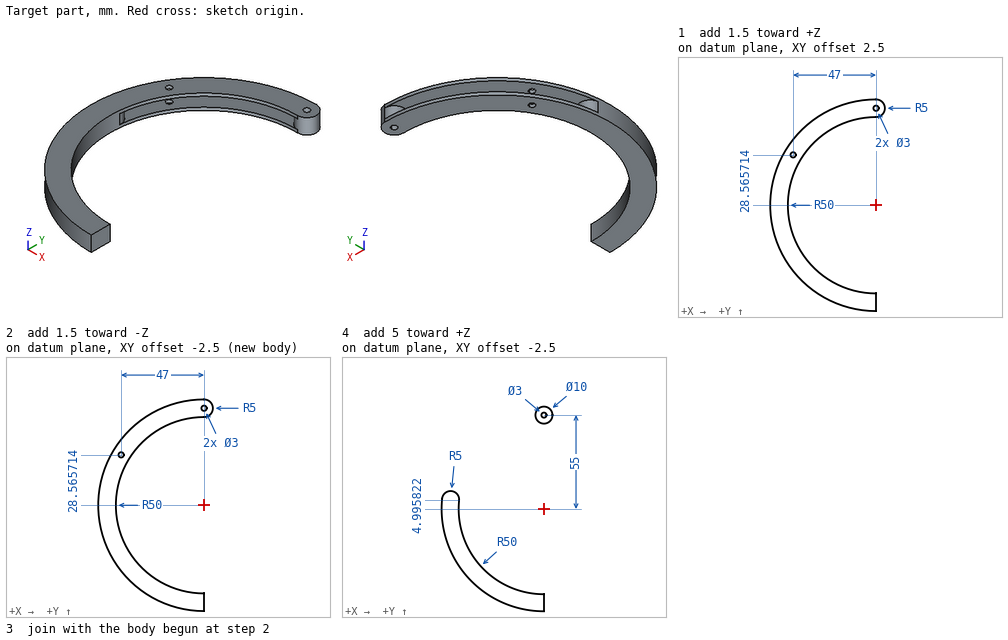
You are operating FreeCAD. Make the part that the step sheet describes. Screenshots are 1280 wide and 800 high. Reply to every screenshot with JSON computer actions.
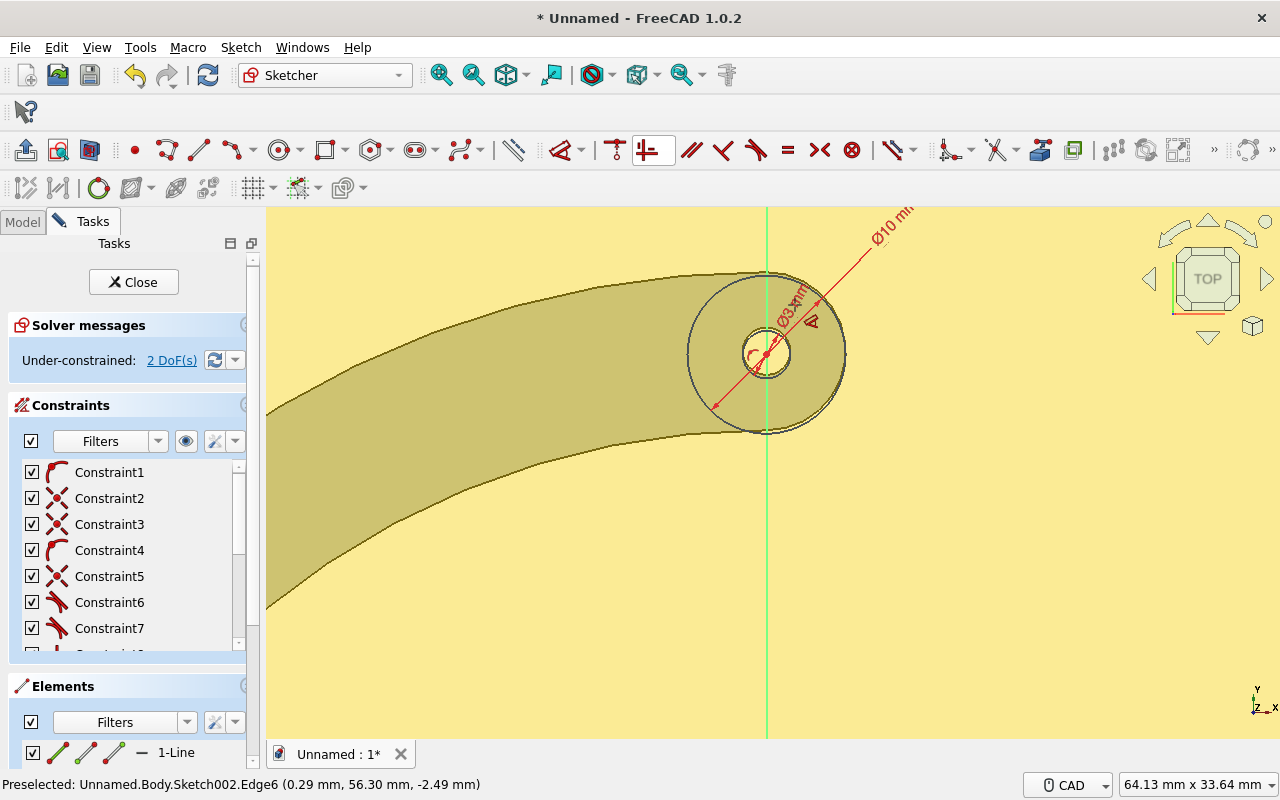
{"action": "scroll", "coordinate": [778, 325], "scroll_direction": "down", "scroll_amount": 9}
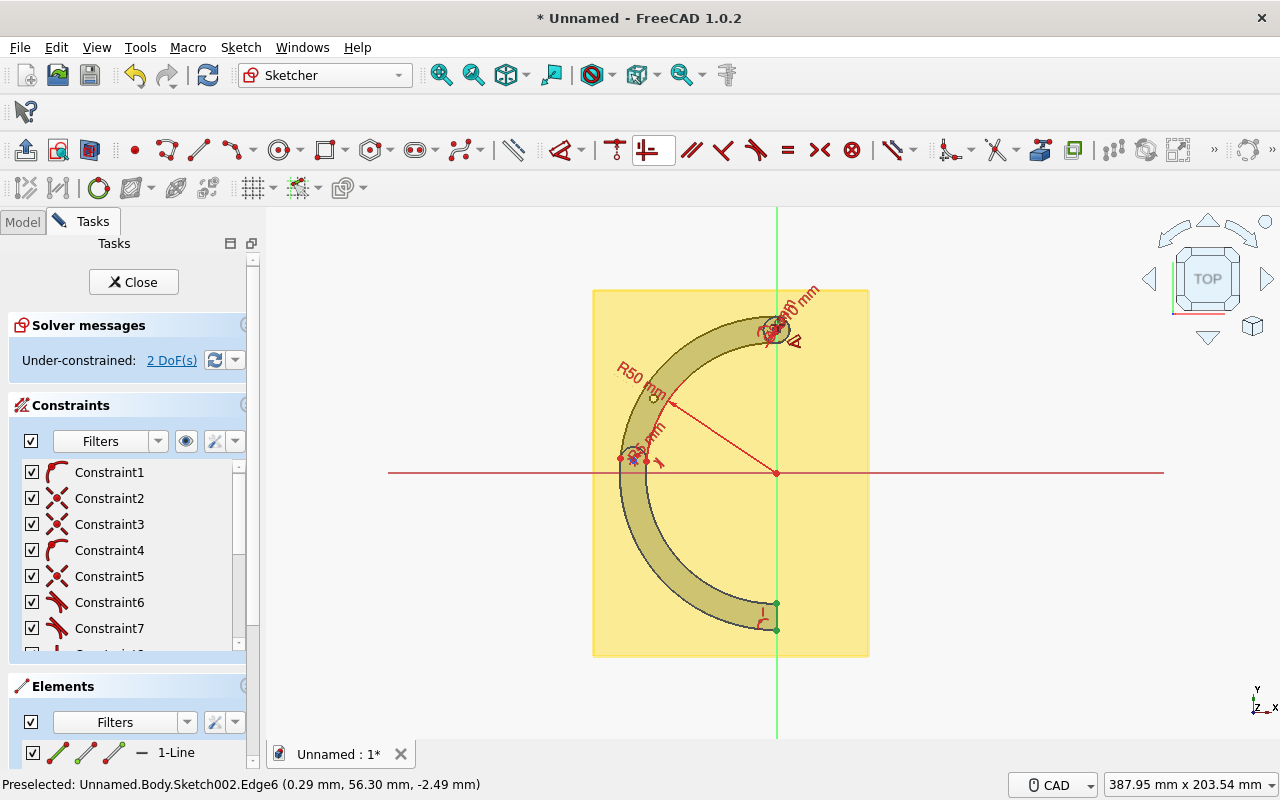
{"action": "left_click", "coordinate": [777, 330]}
{"action": "left_click", "coordinate": [811, 402]}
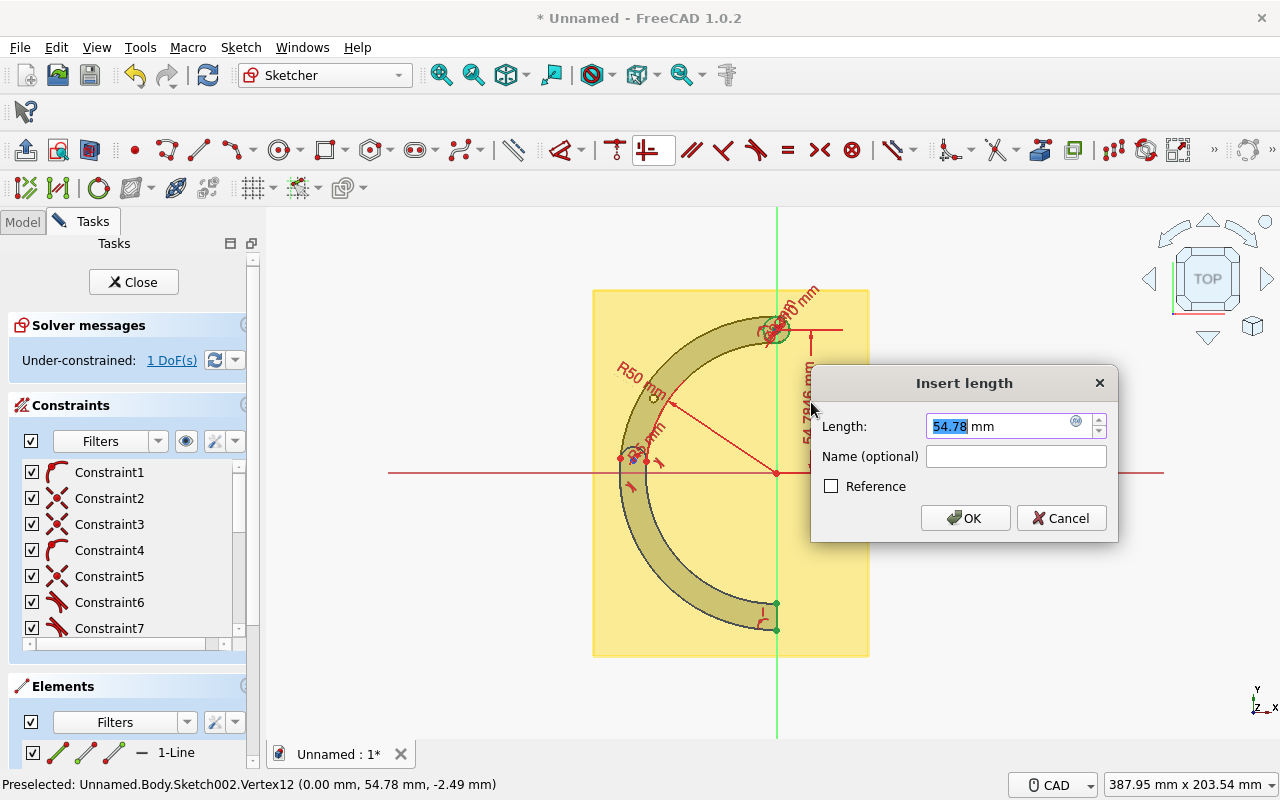
{"action": "type", "text": "55"}
{"action": "key", "text": "Return"}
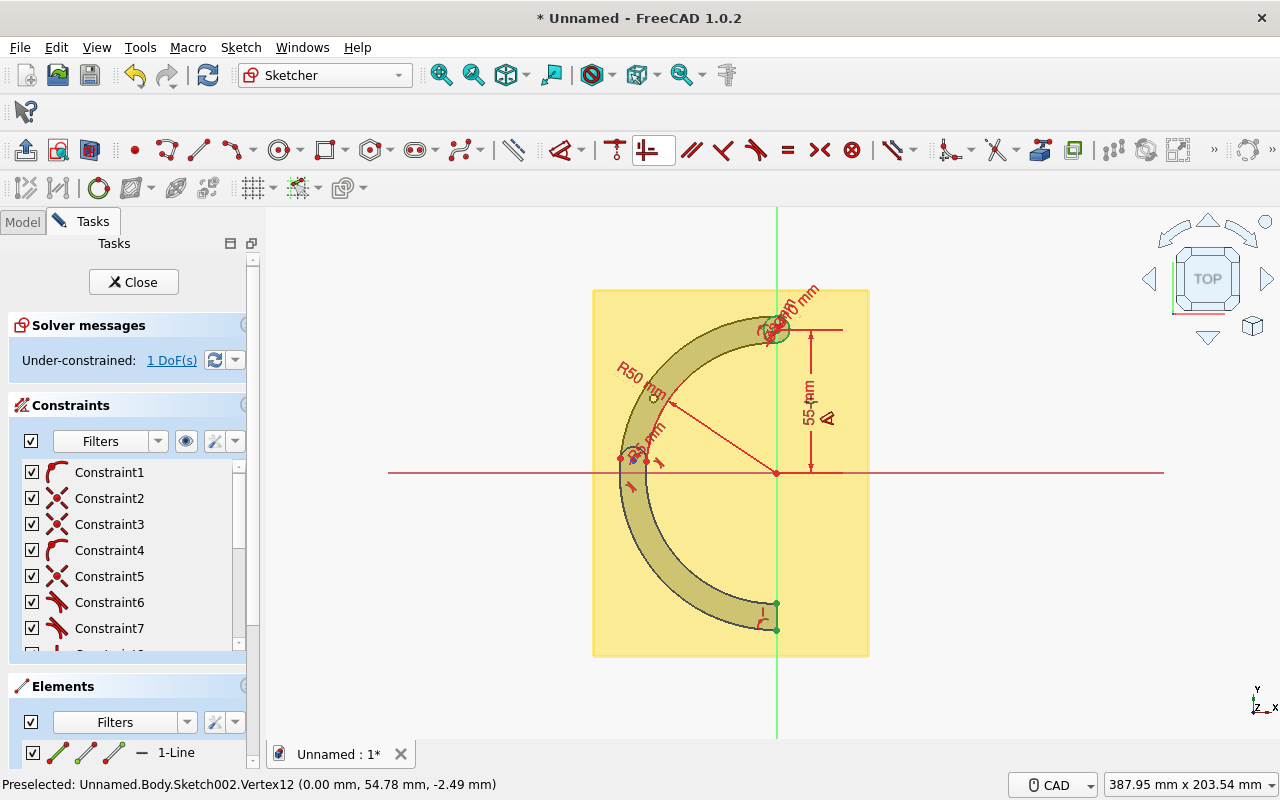
{"action": "scroll", "coordinate": [646, 461], "scroll_direction": "up", "scroll_amount": 6}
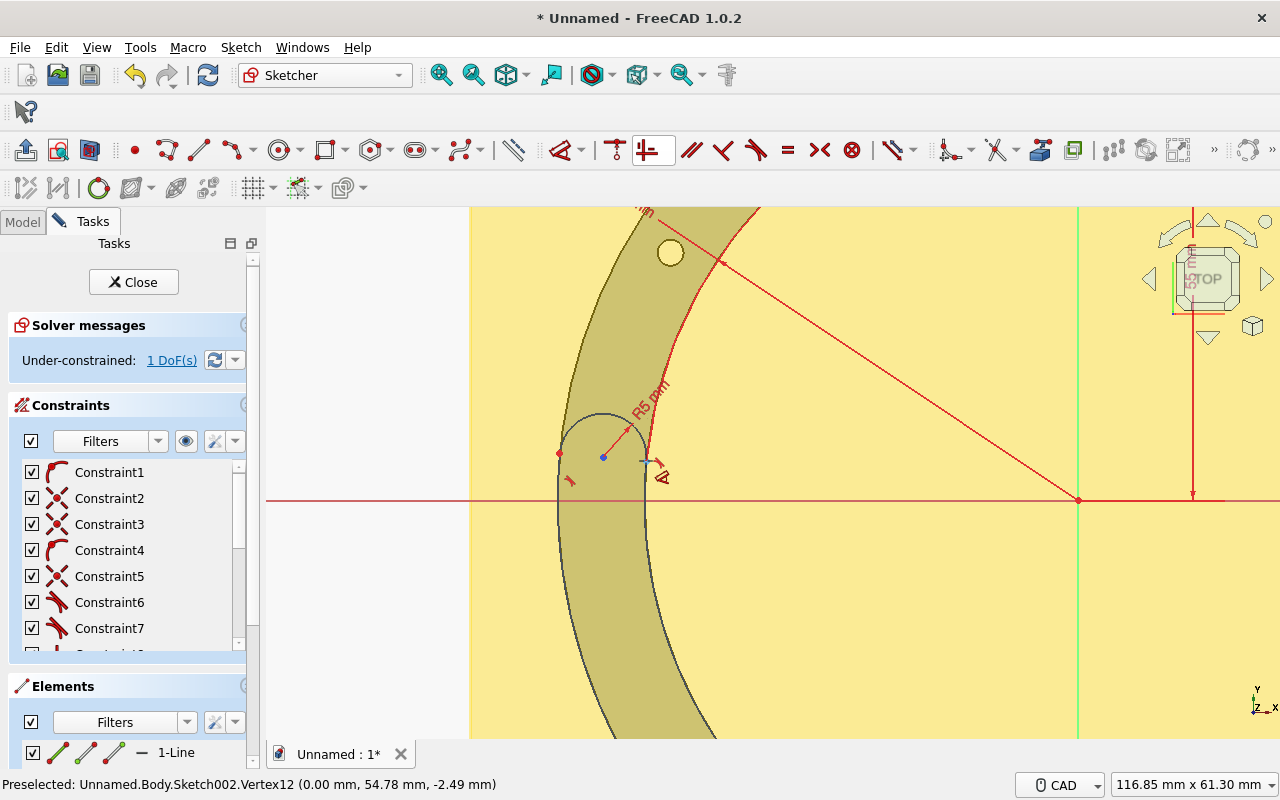
{"action": "left_click", "coordinate": [646, 461]}
{"action": "left_click", "coordinate": [1112, 481]}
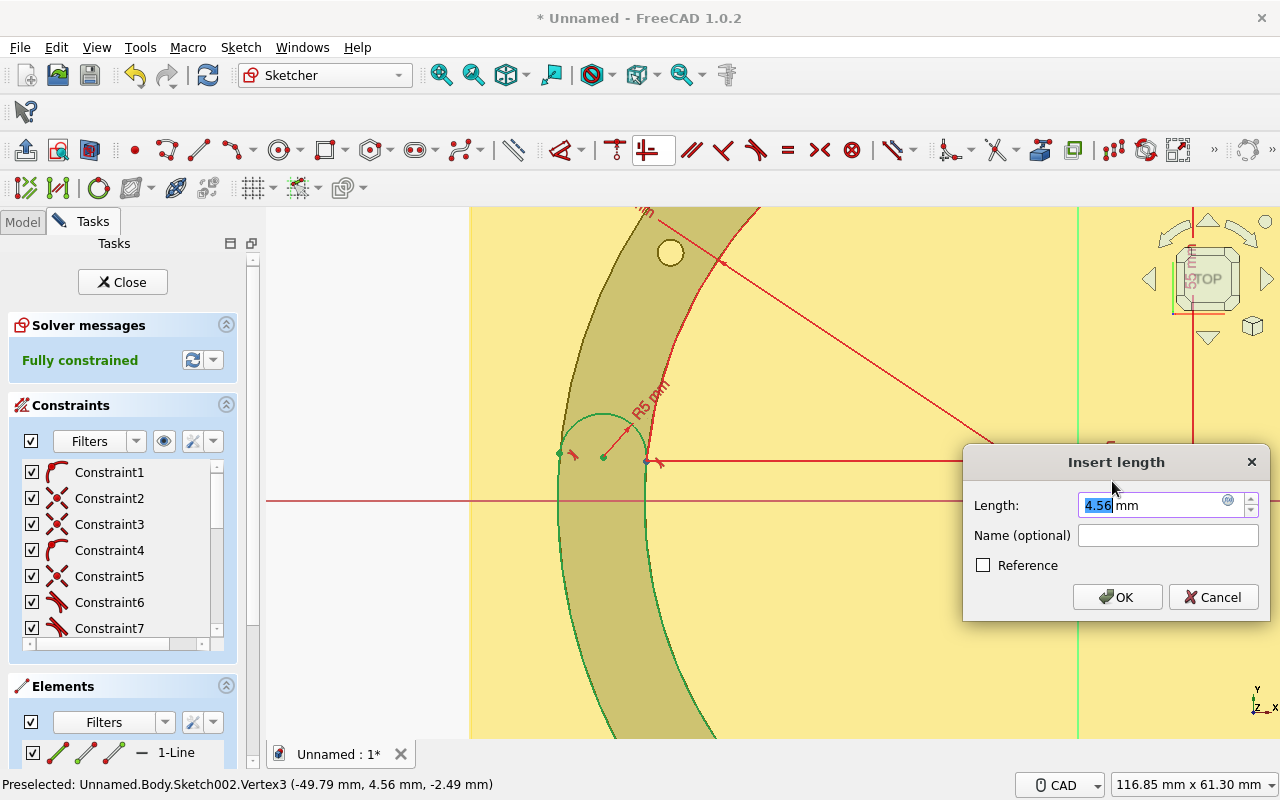
{"action": "type", "text": "4.995822"}
{"action": "key", "text": "Return"}
{"action": "key", "text": "Escape"}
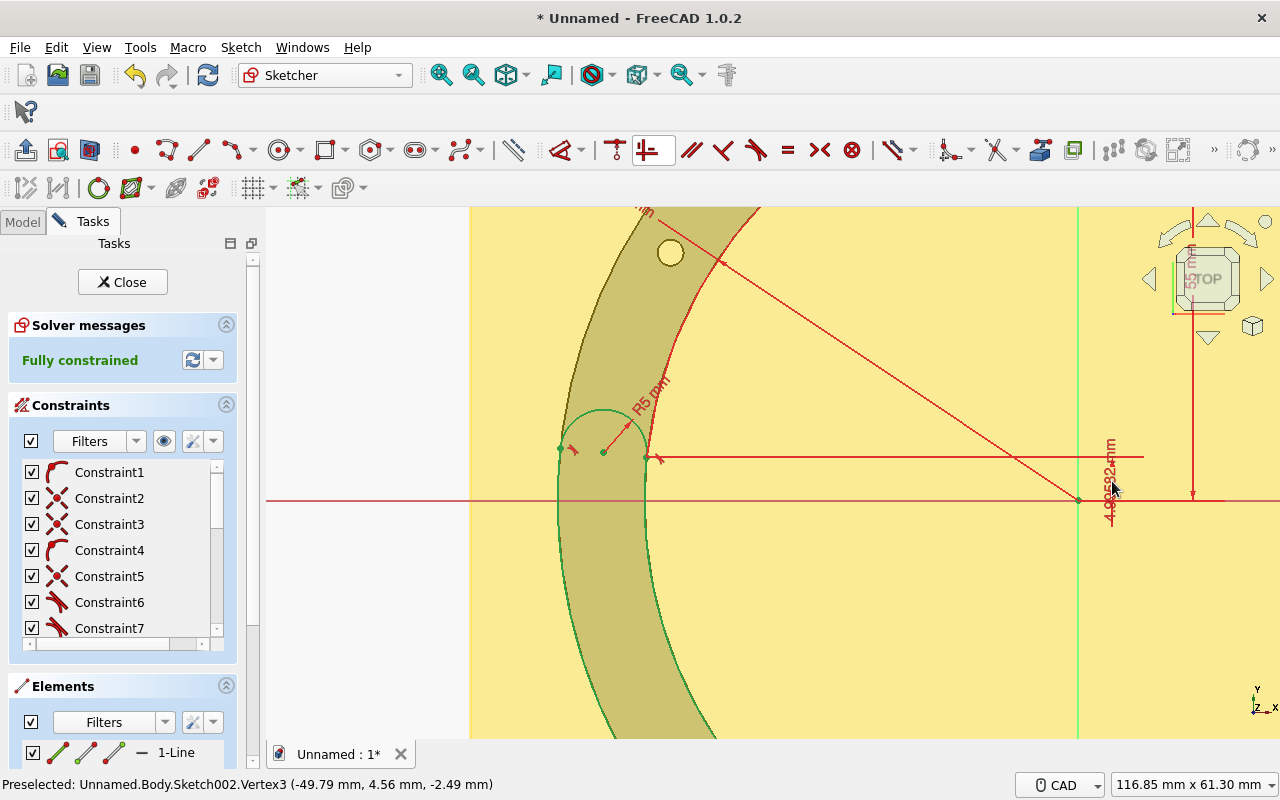
{"action": "left_click", "coordinate": [123, 282]}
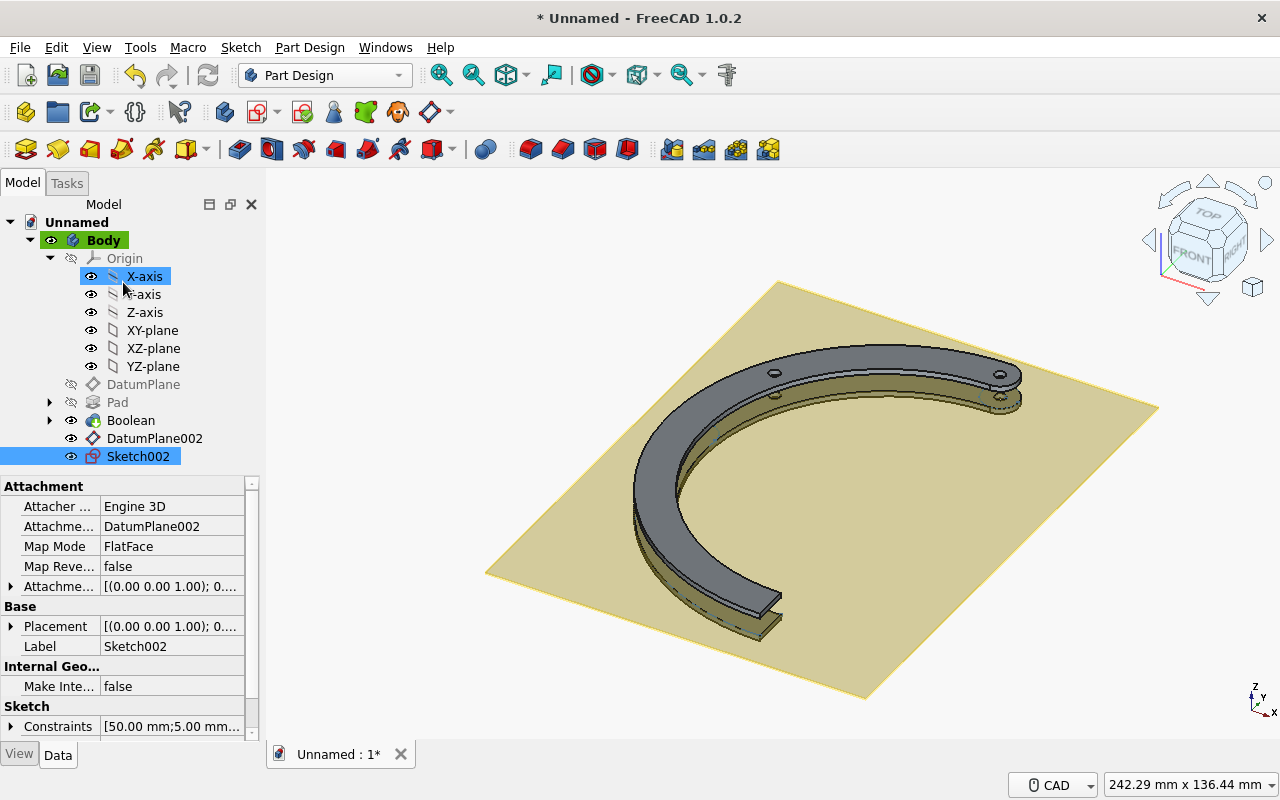
{"action": "left_click", "coordinate": [26, 150]}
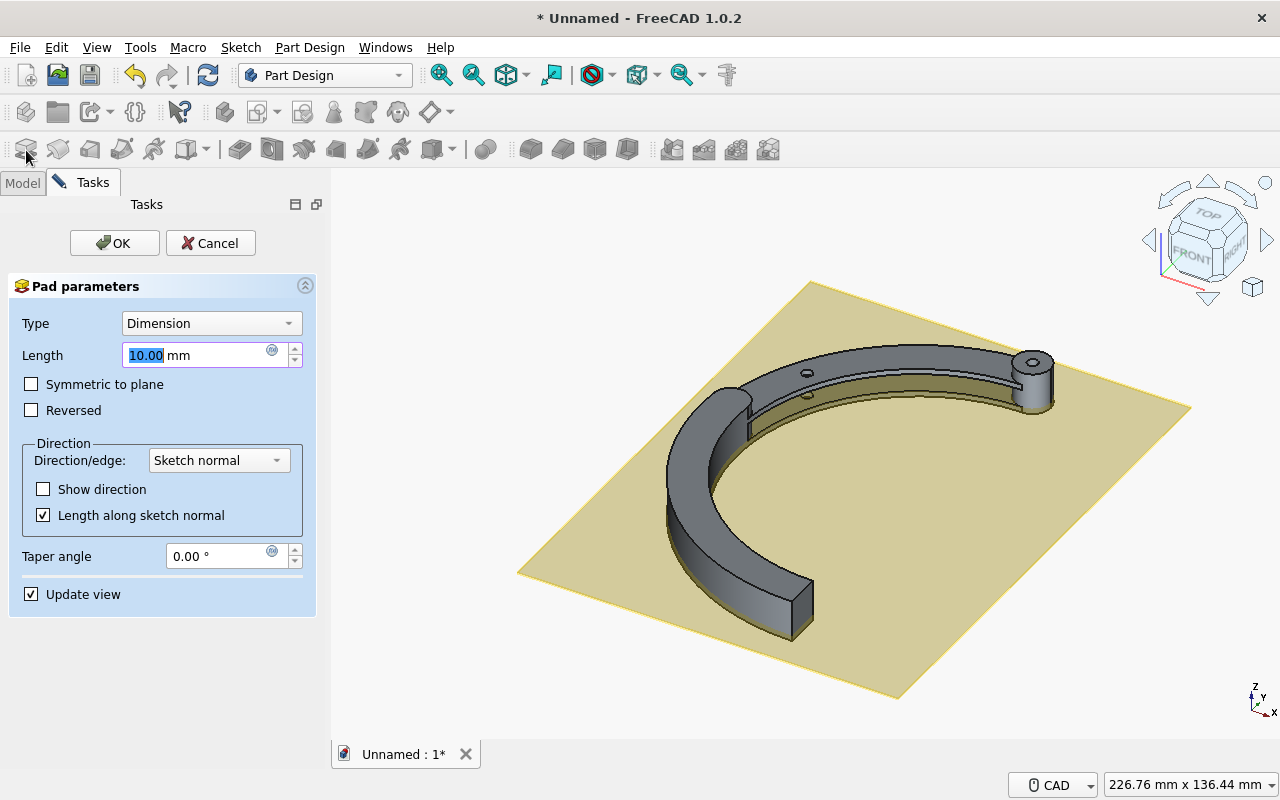
{"action": "type", "text": "5"}
{"action": "key", "text": "Tab"}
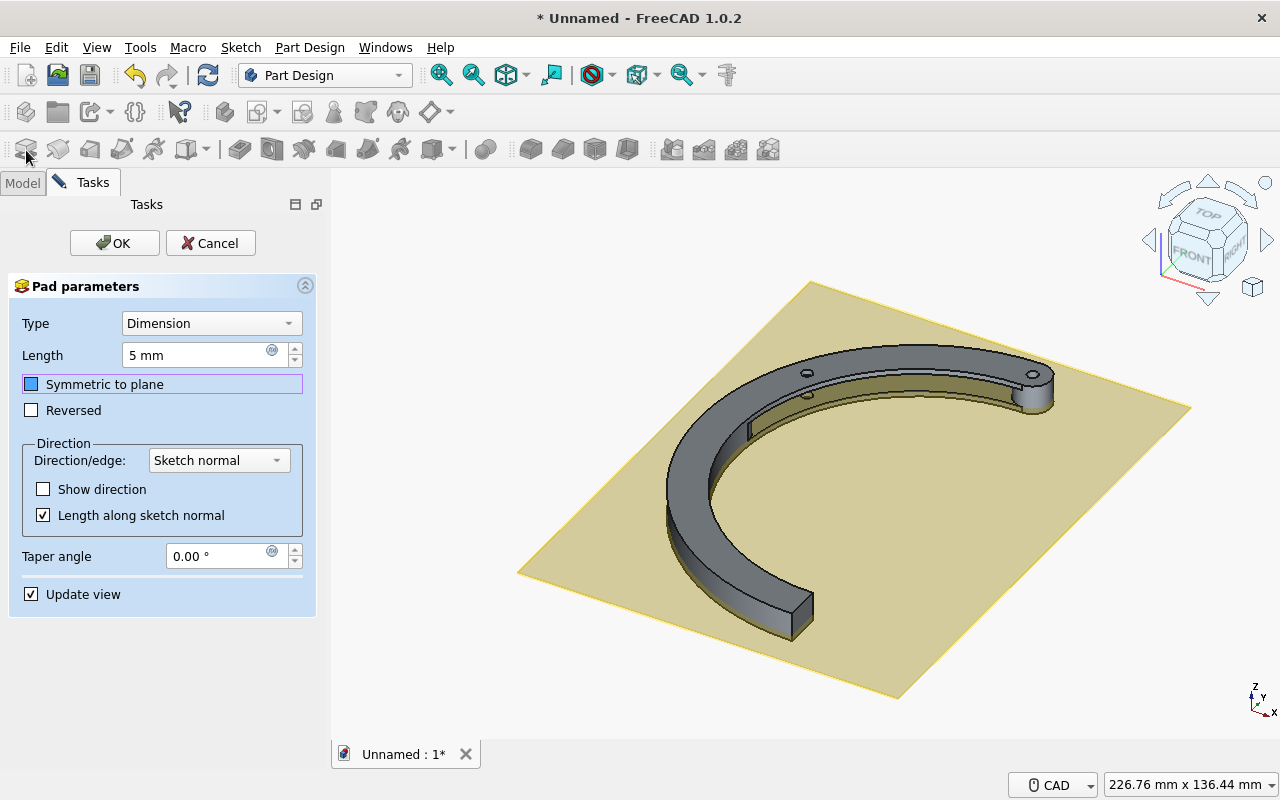
{"action": "left_click", "coordinate": [115, 243]}